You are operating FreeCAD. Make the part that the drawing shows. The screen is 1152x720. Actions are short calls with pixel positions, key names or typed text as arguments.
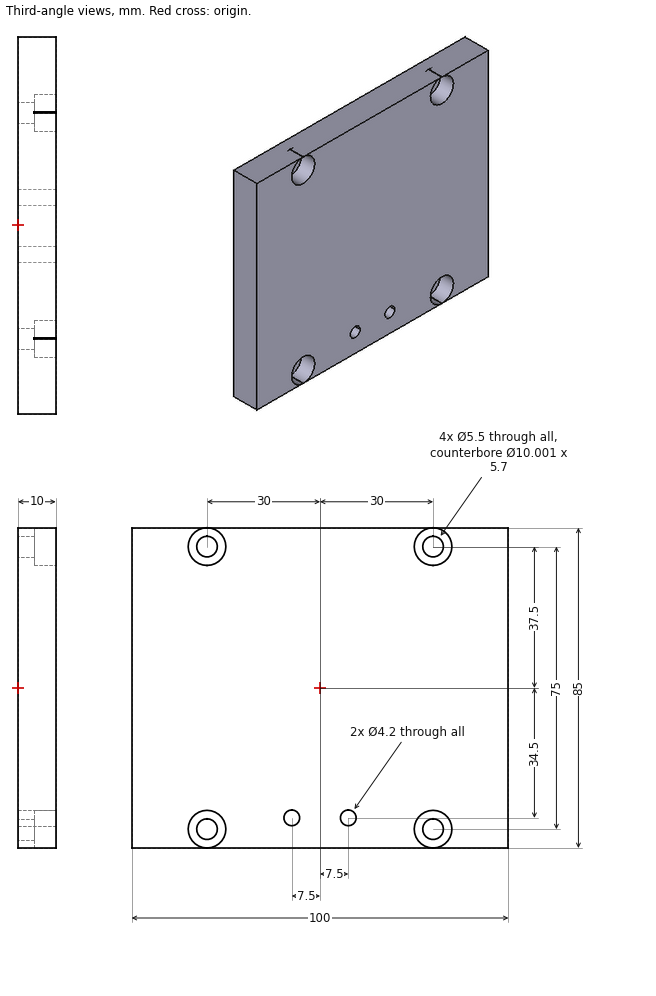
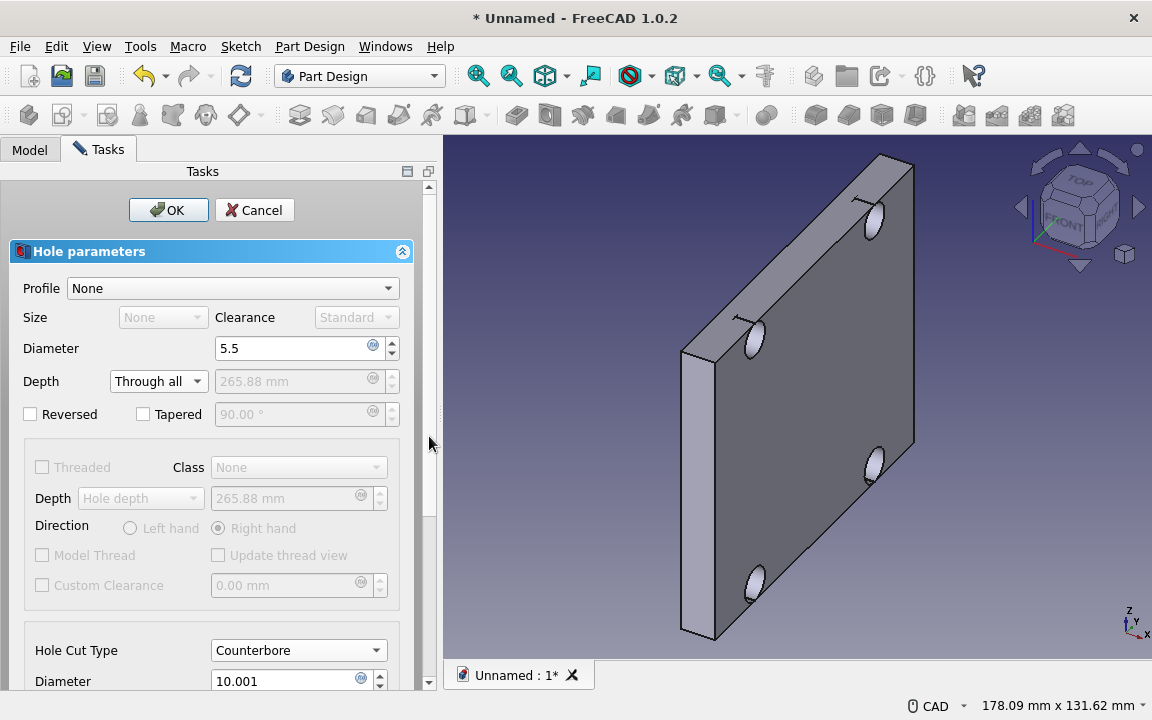
click(169, 210)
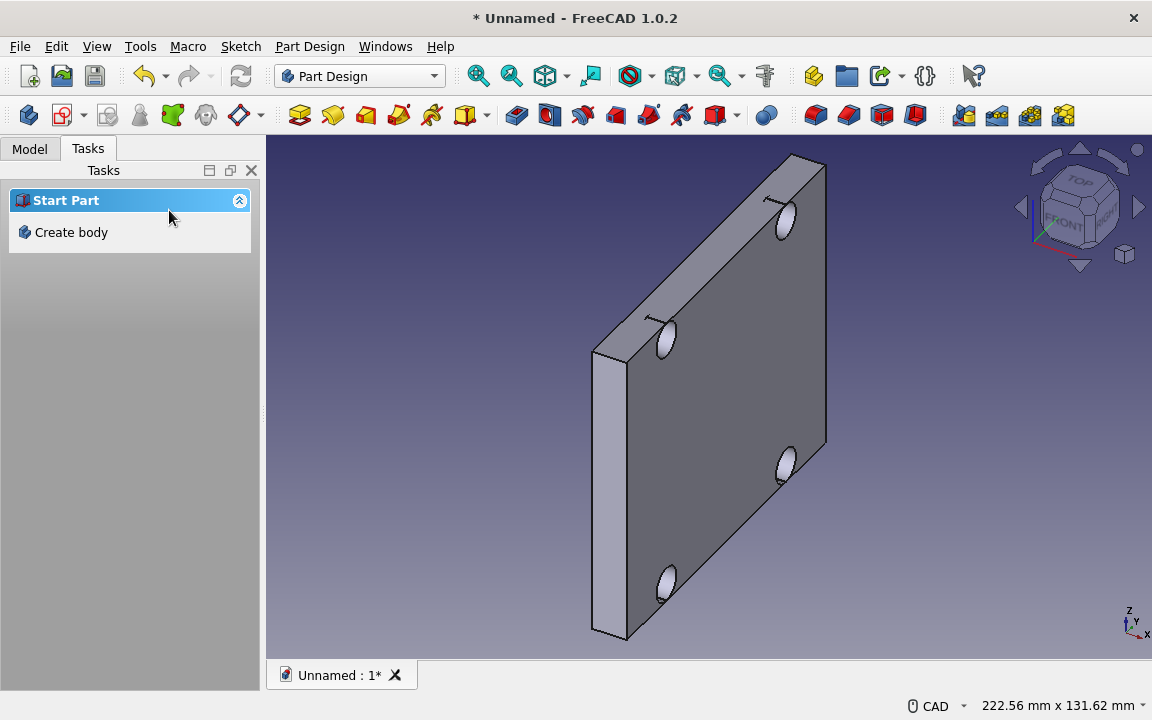
click(726, 402)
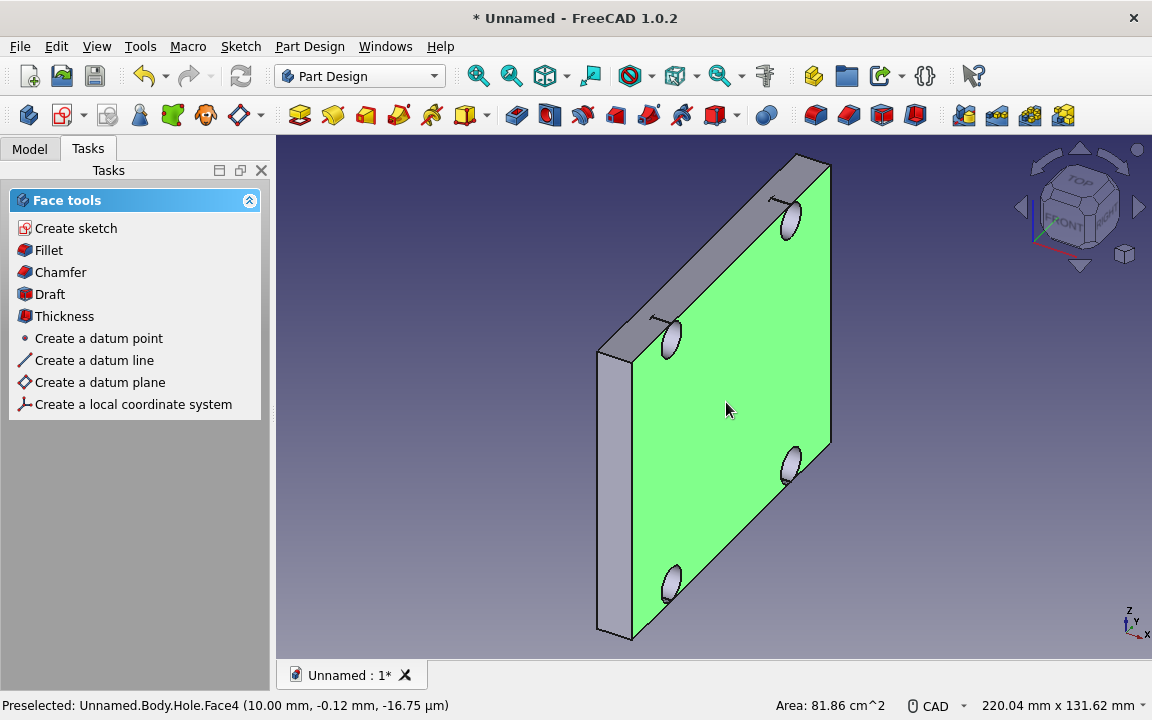
click(62, 116)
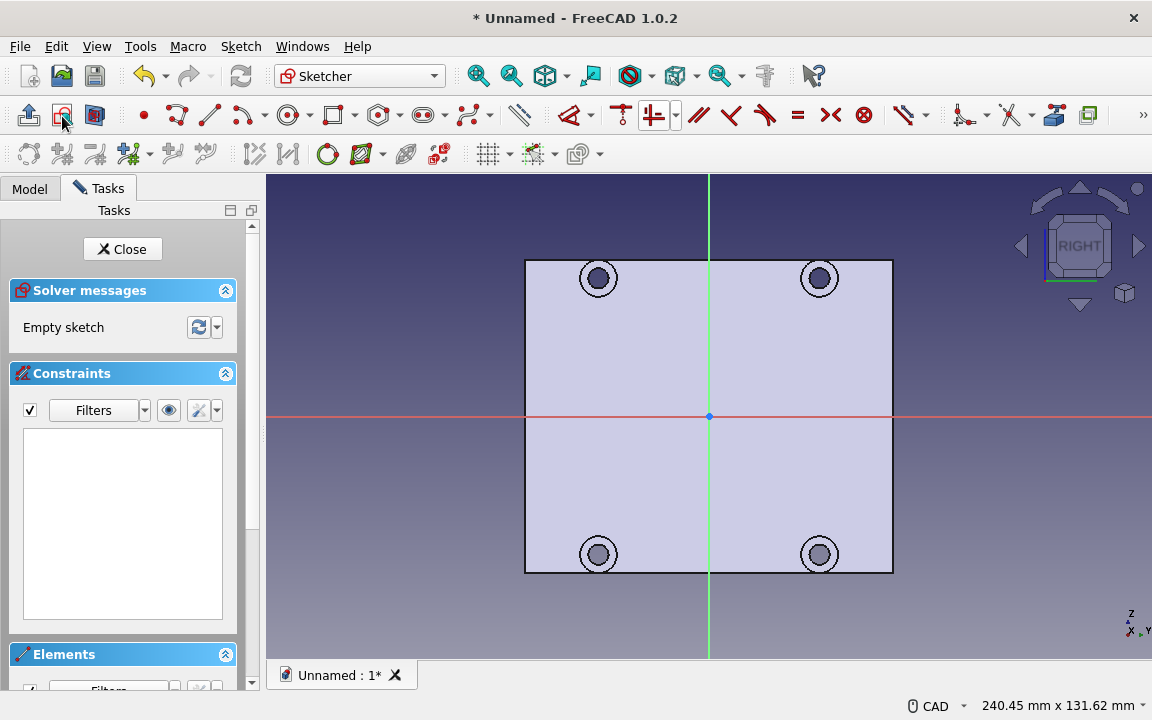
scroll(765, 539, up, 4)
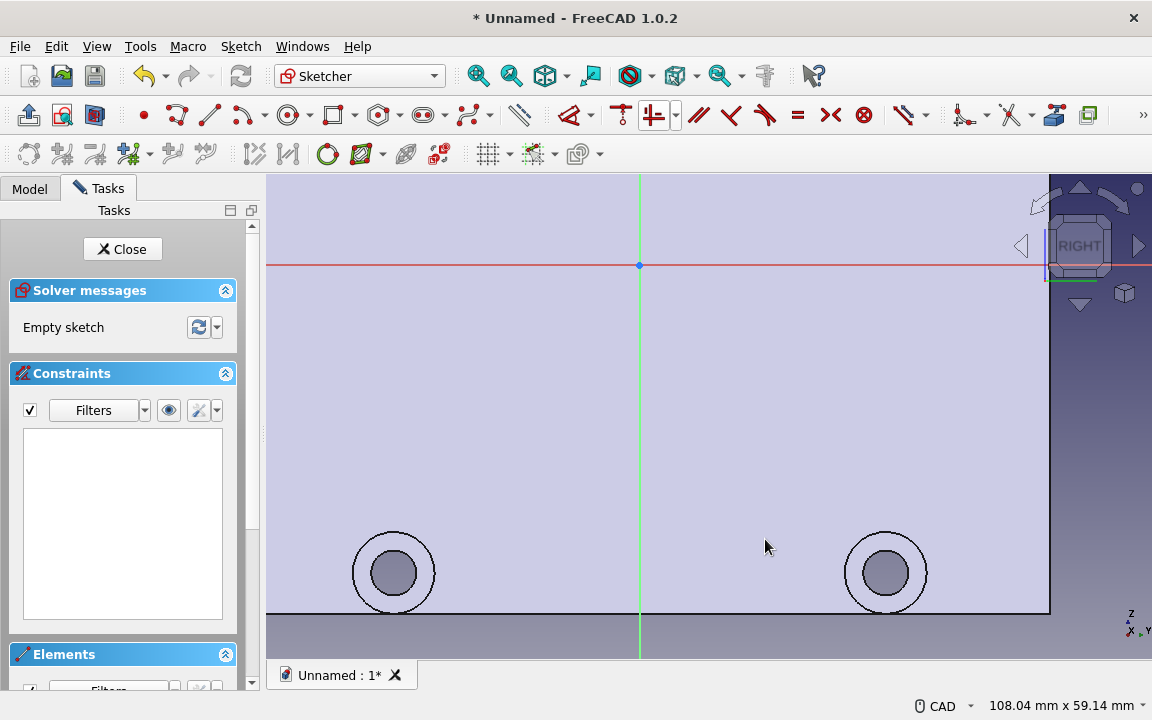
click(288, 116)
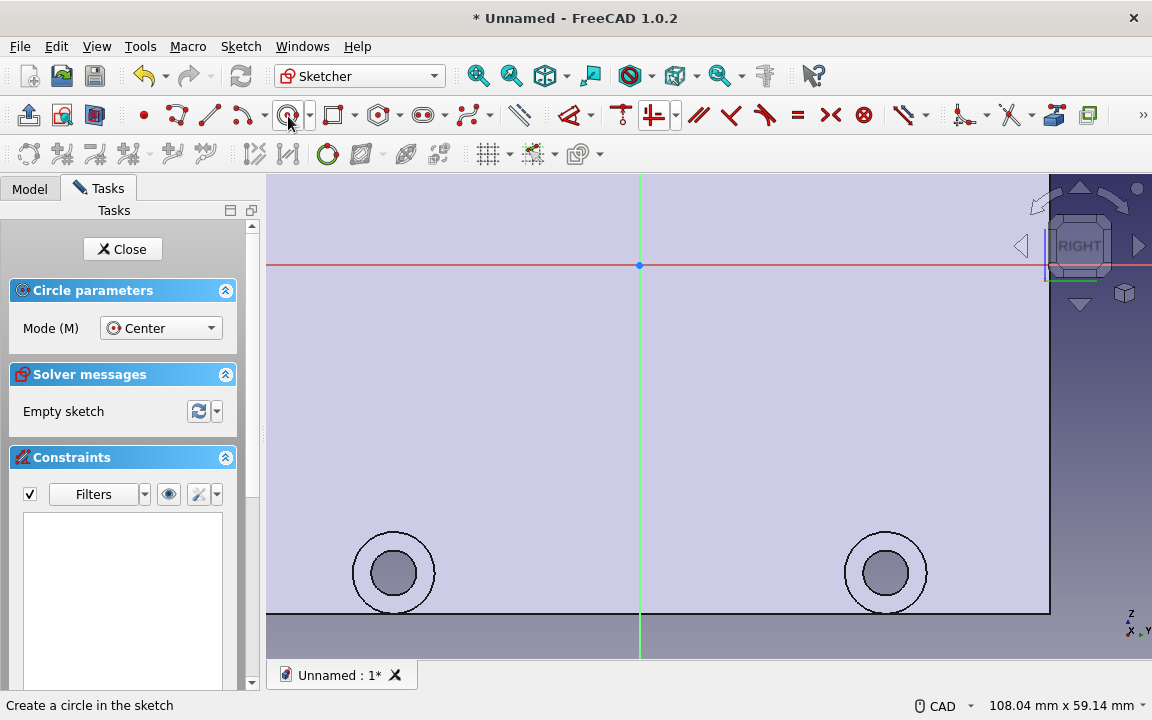
scroll(701, 548, up, 2)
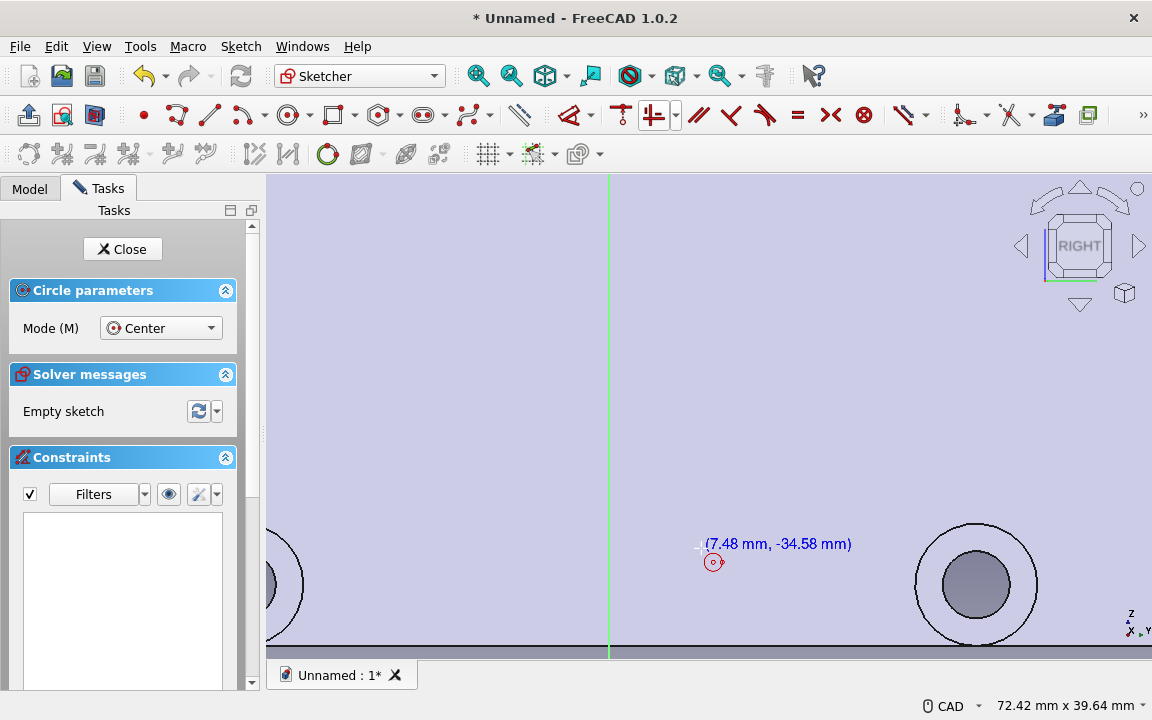
click(701, 548)
click(719, 530)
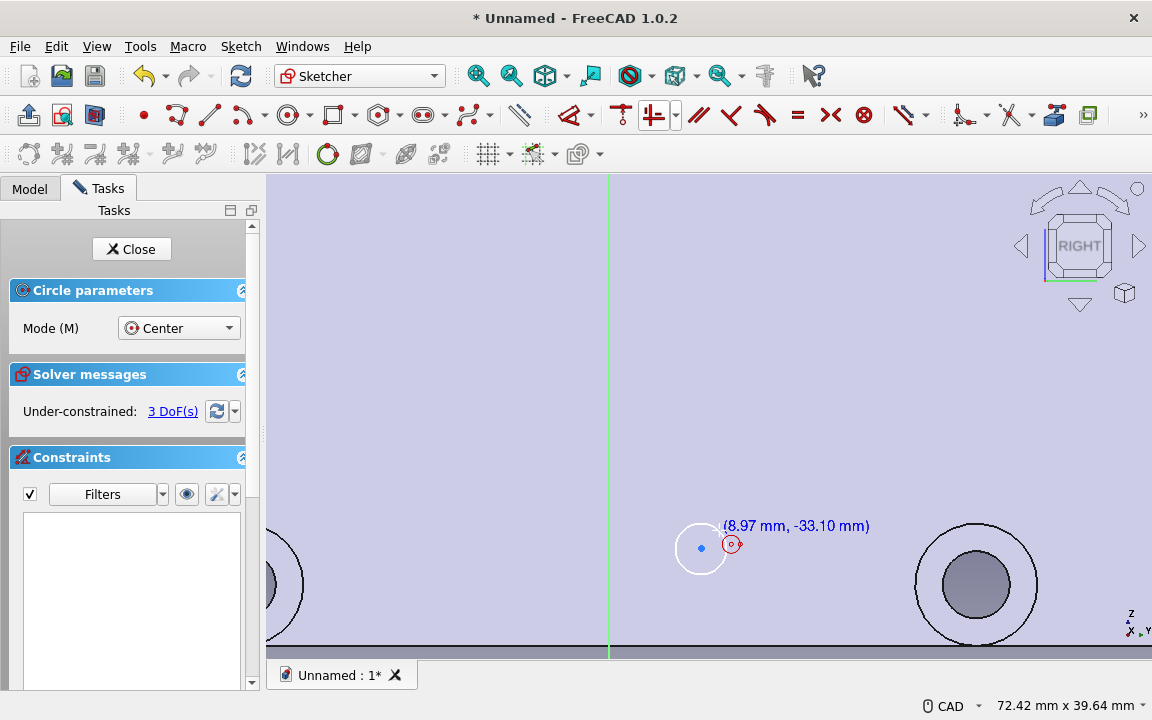
click(518, 548)
click(536, 530)
key(Escape)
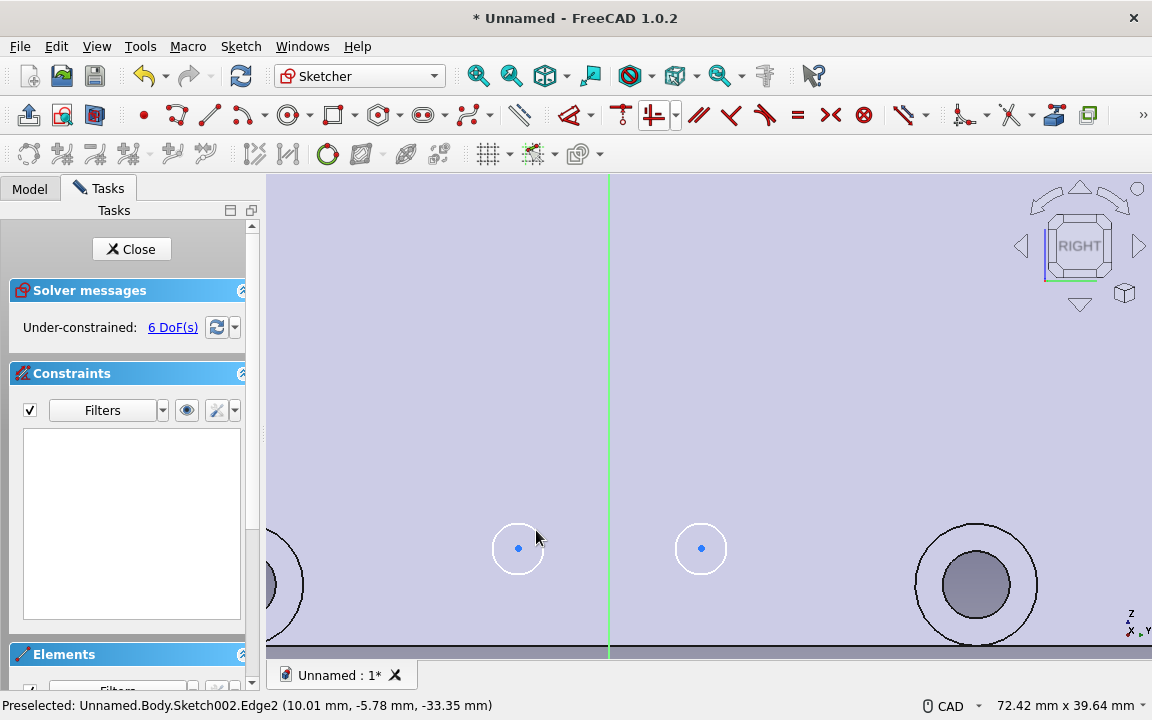
click(719, 531)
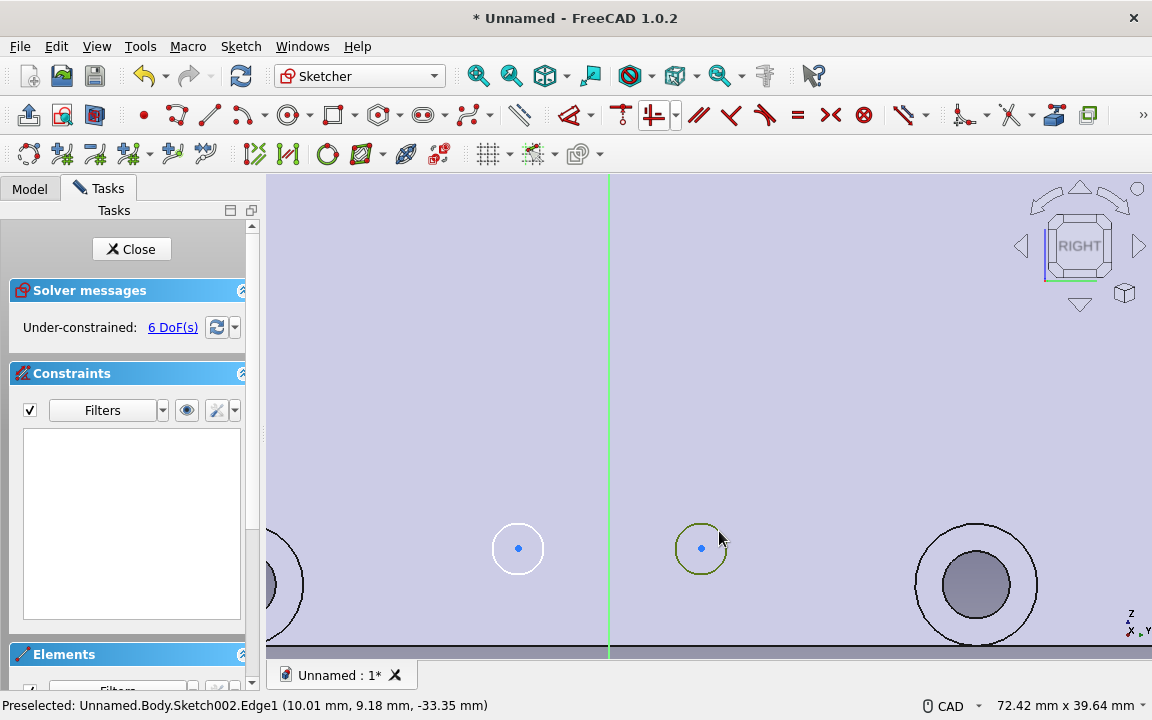
click(536, 531)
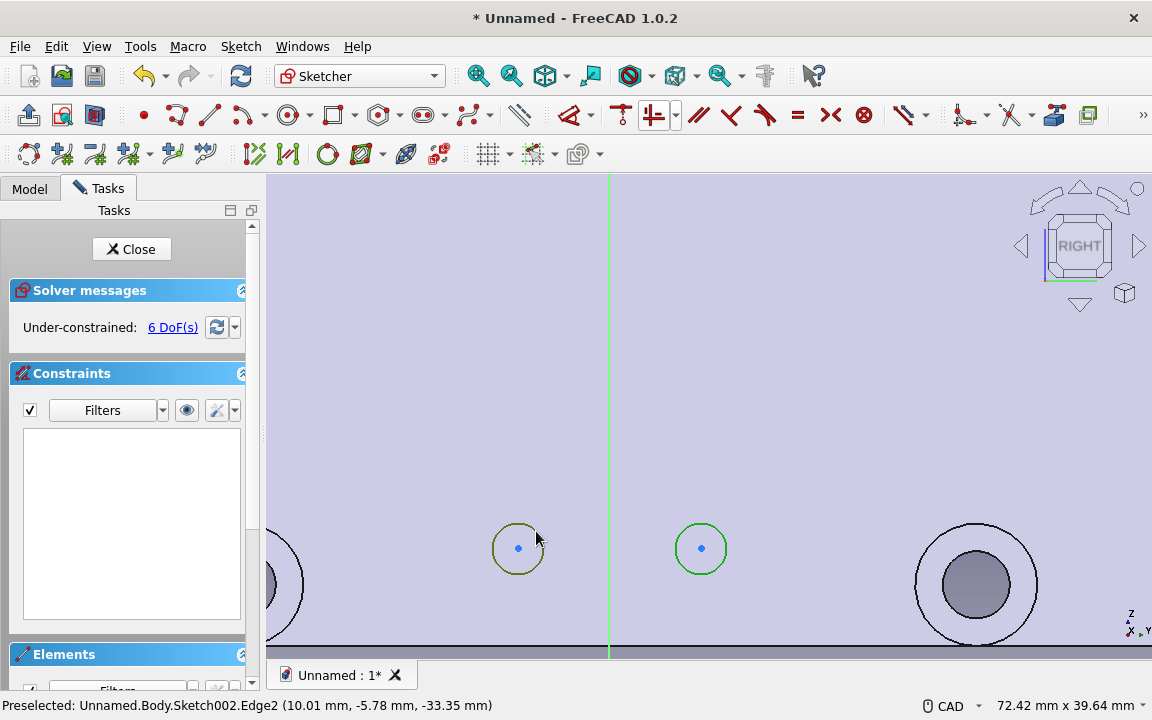
click(798, 116)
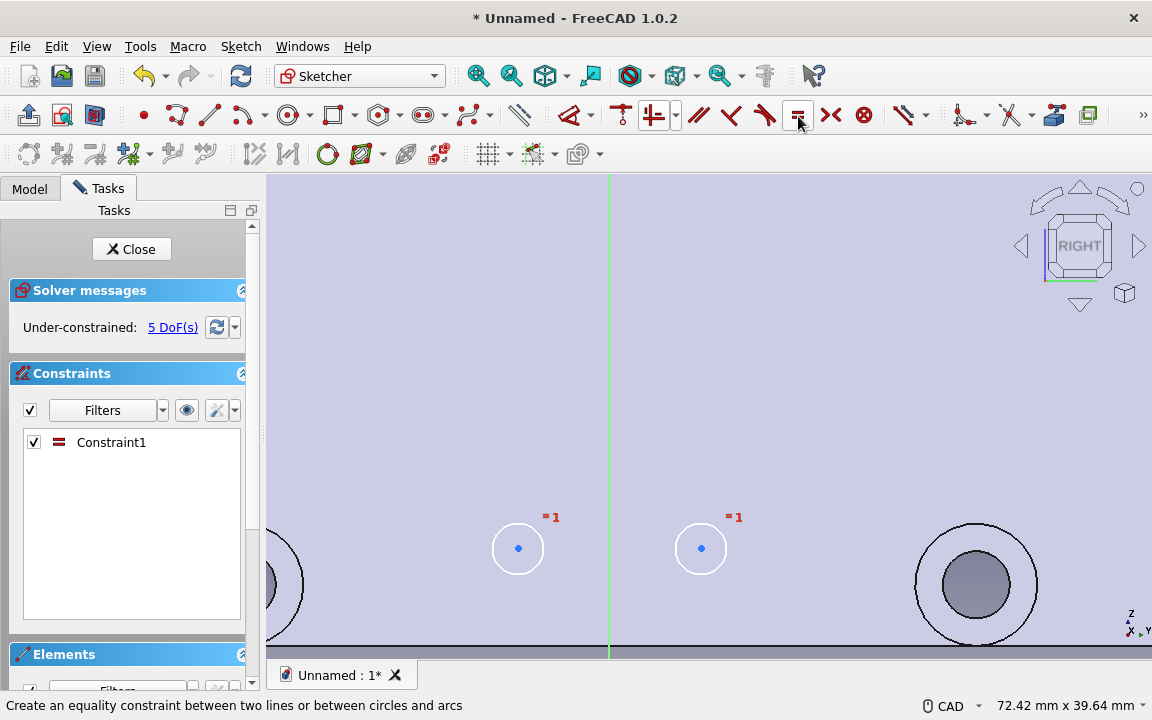
click(701, 549)